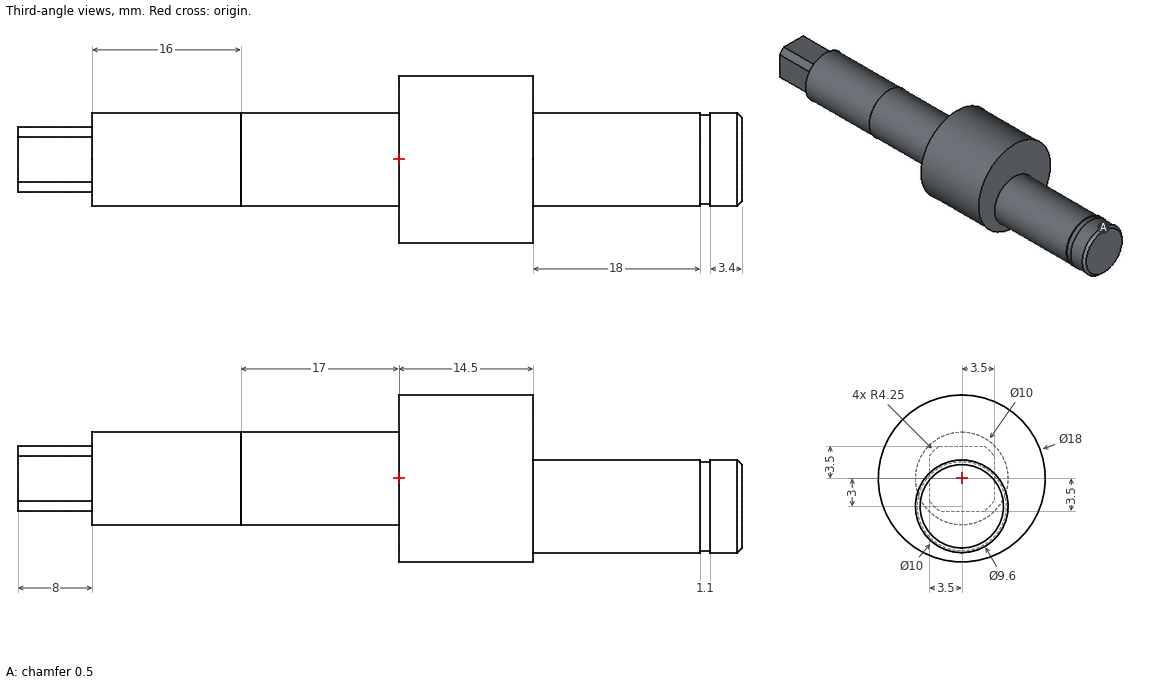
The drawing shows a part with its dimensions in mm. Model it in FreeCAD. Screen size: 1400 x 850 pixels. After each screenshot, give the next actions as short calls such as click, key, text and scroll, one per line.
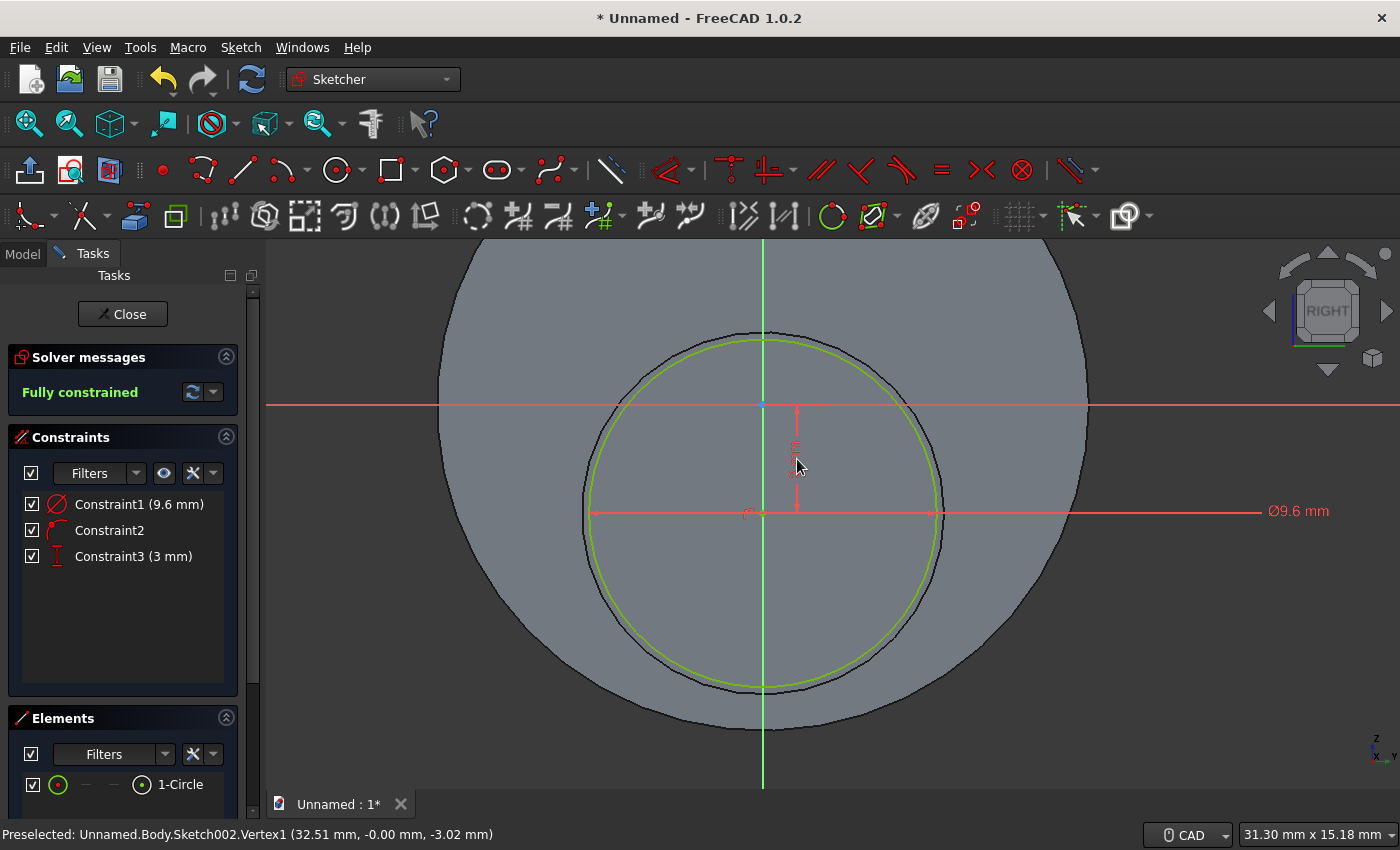
click(123, 314)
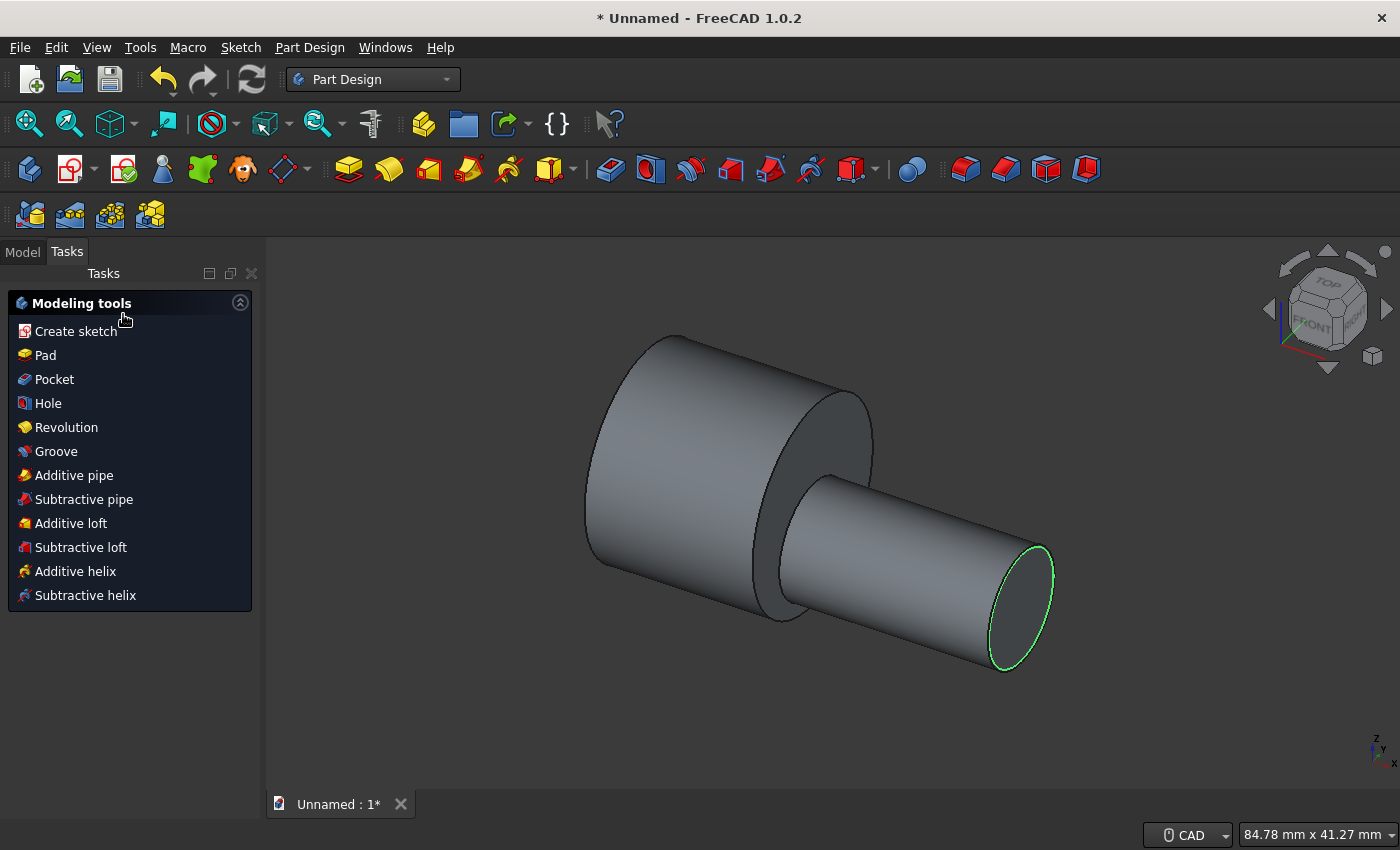
click(350, 170)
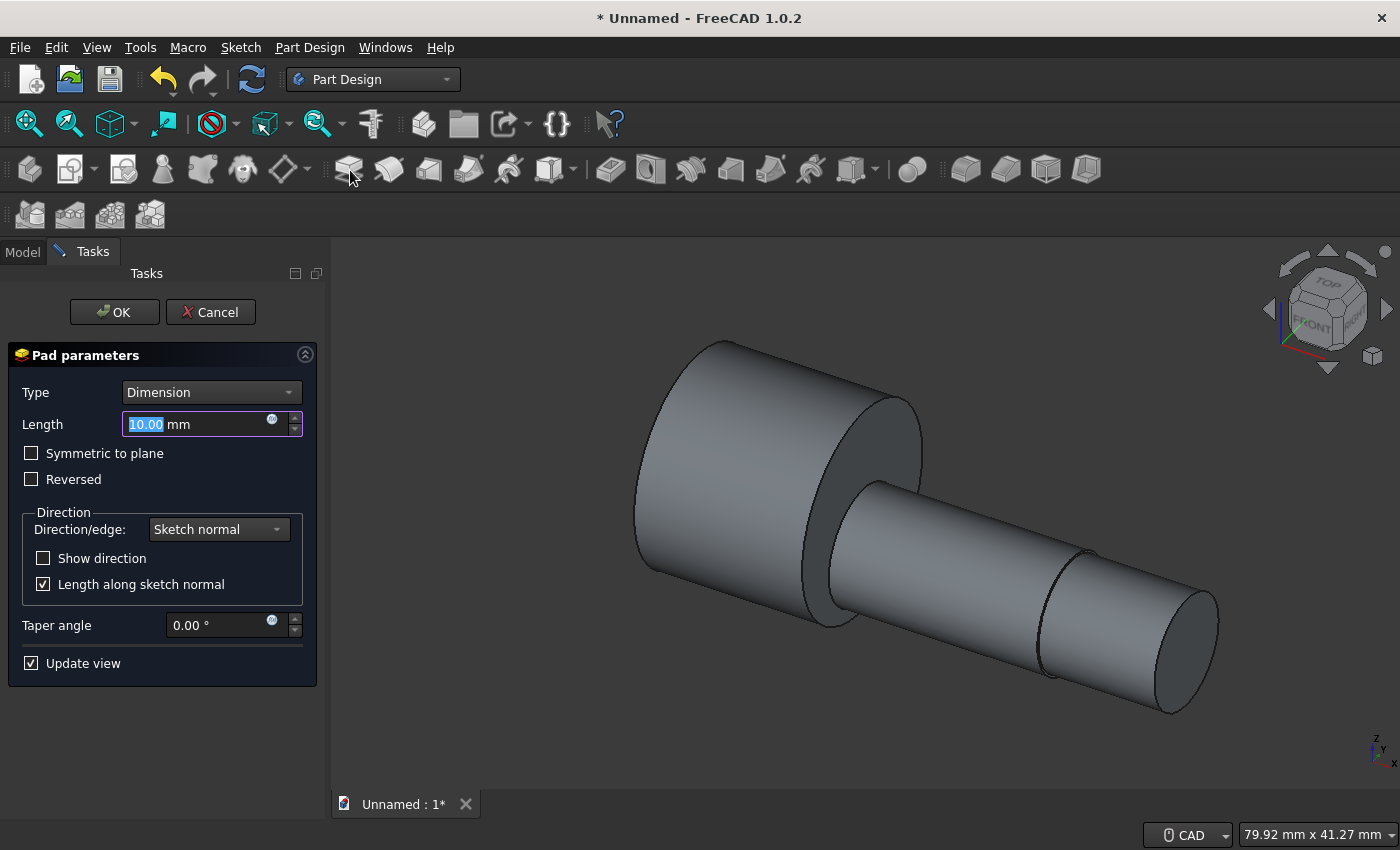
text(1.1)
key(Tab)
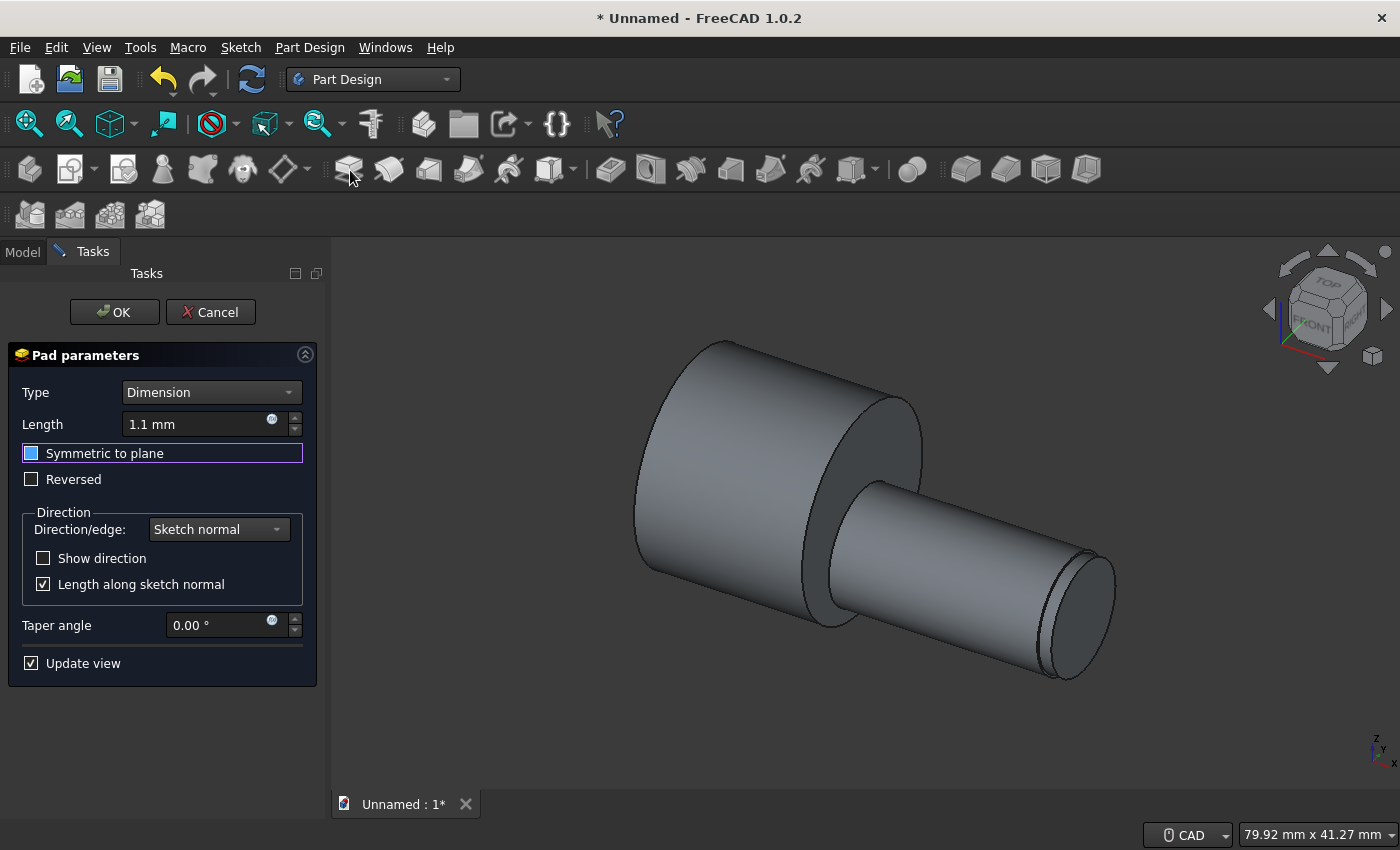
click(115, 312)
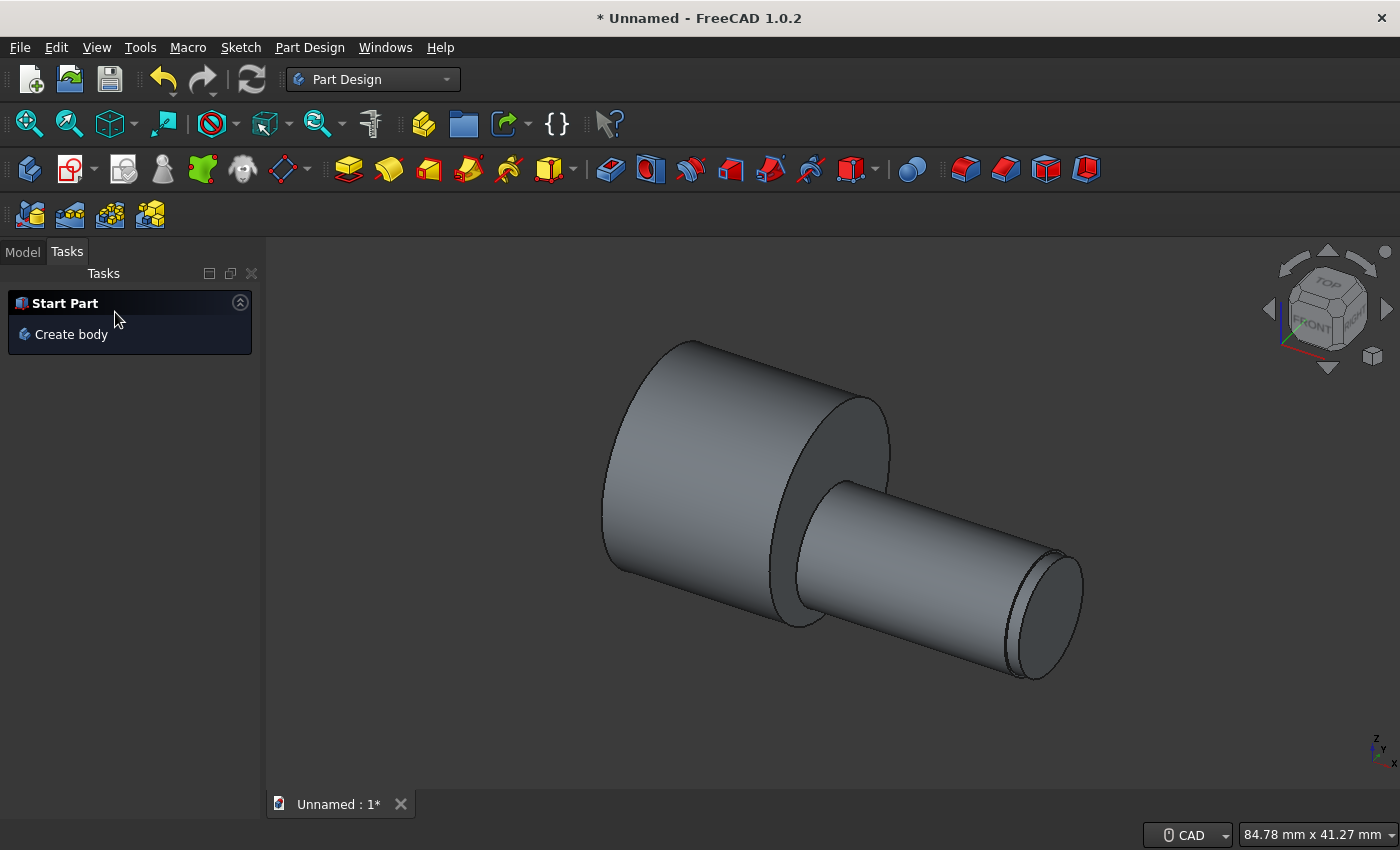
click(1051, 617)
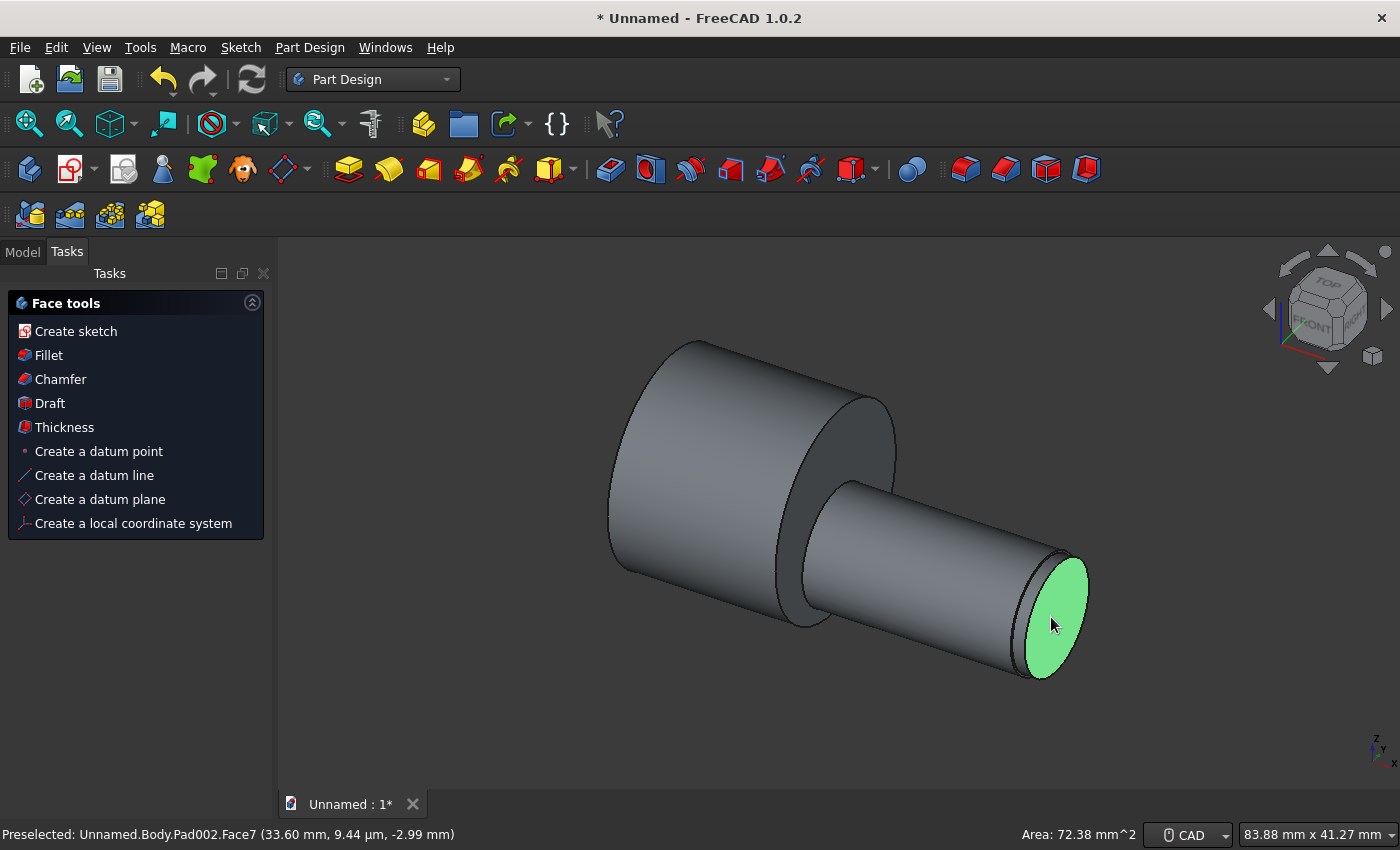
click(70, 170)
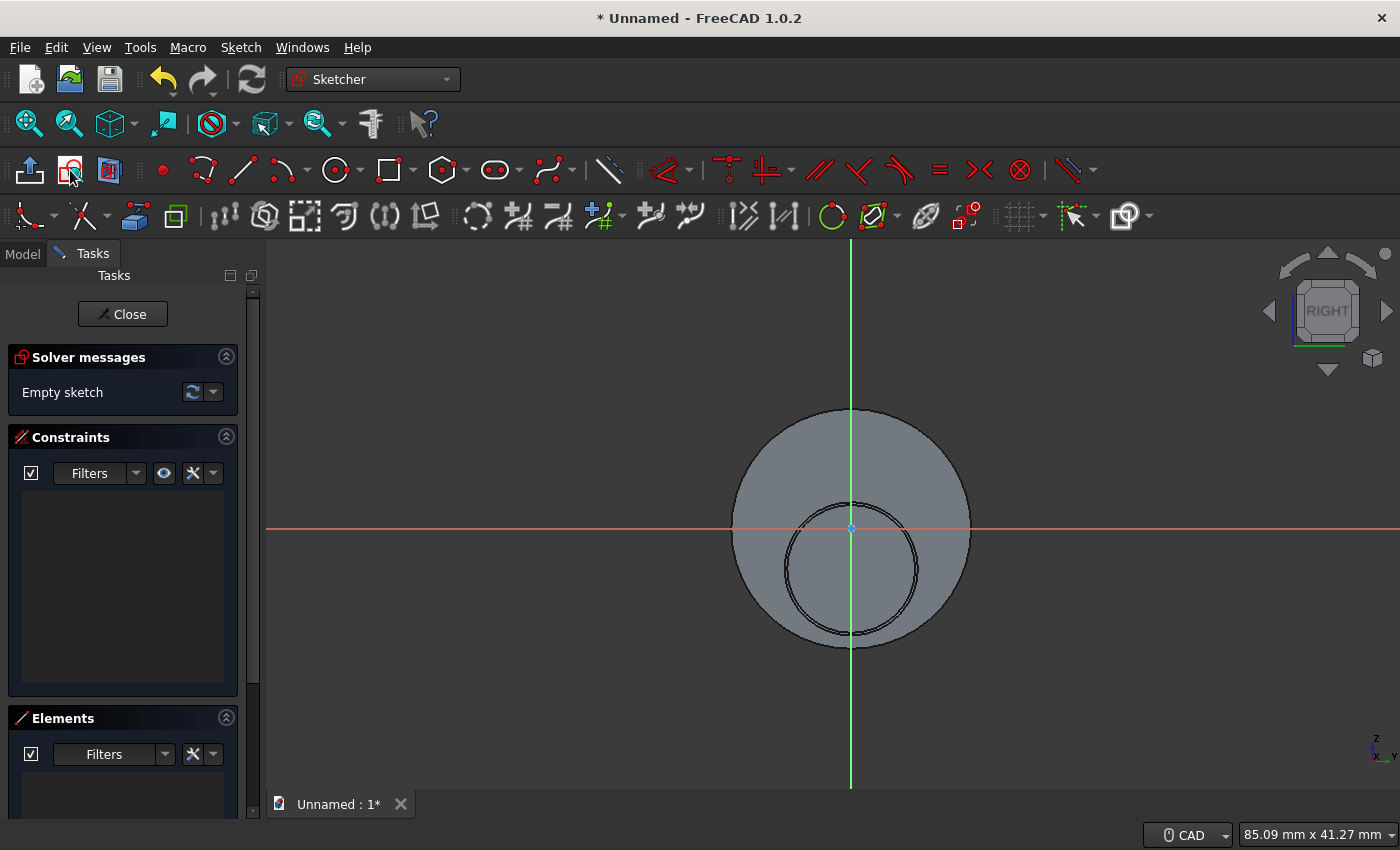
scroll(902, 601, up, 5)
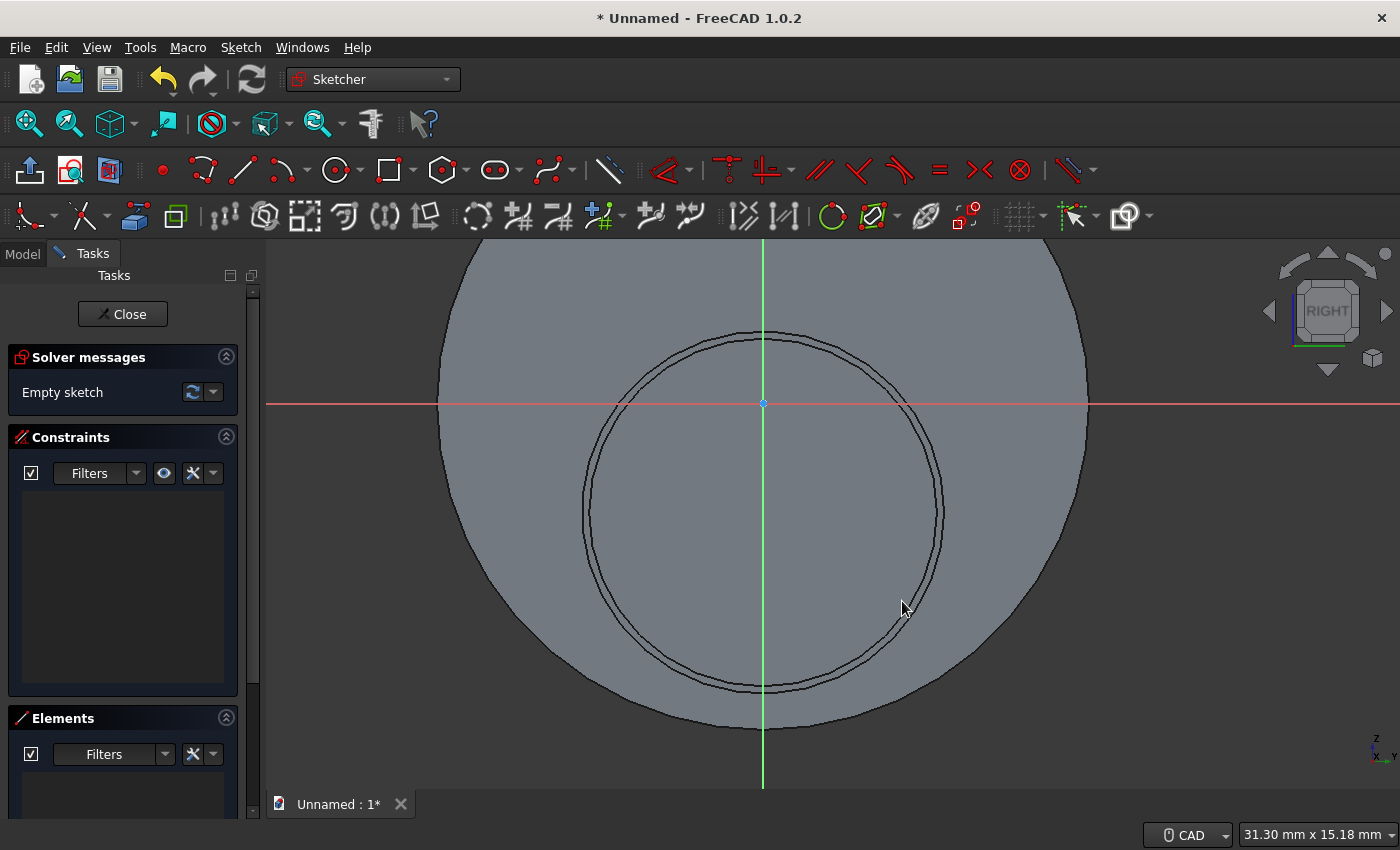
click(336, 170)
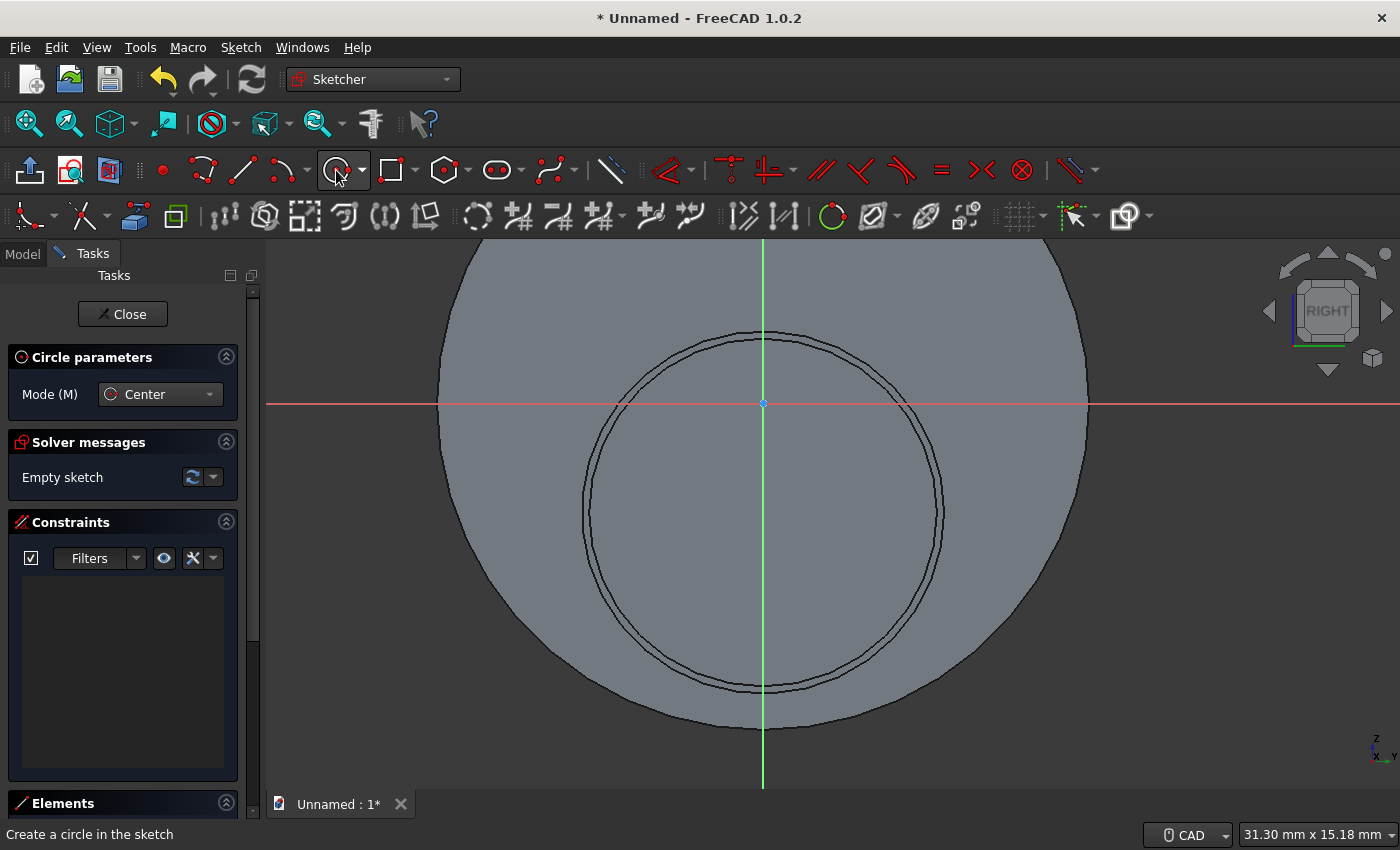
click(763, 513)
move(891, 384)